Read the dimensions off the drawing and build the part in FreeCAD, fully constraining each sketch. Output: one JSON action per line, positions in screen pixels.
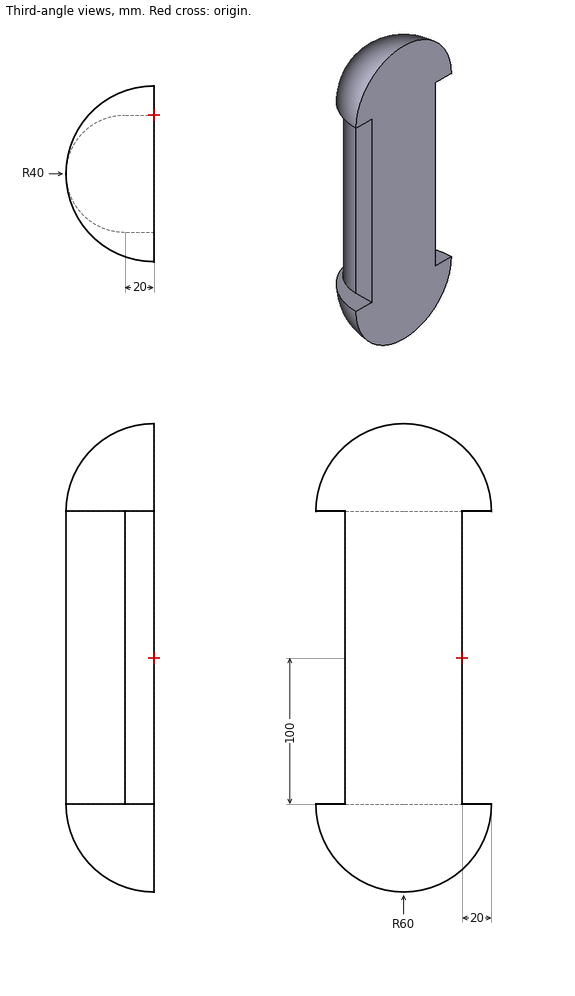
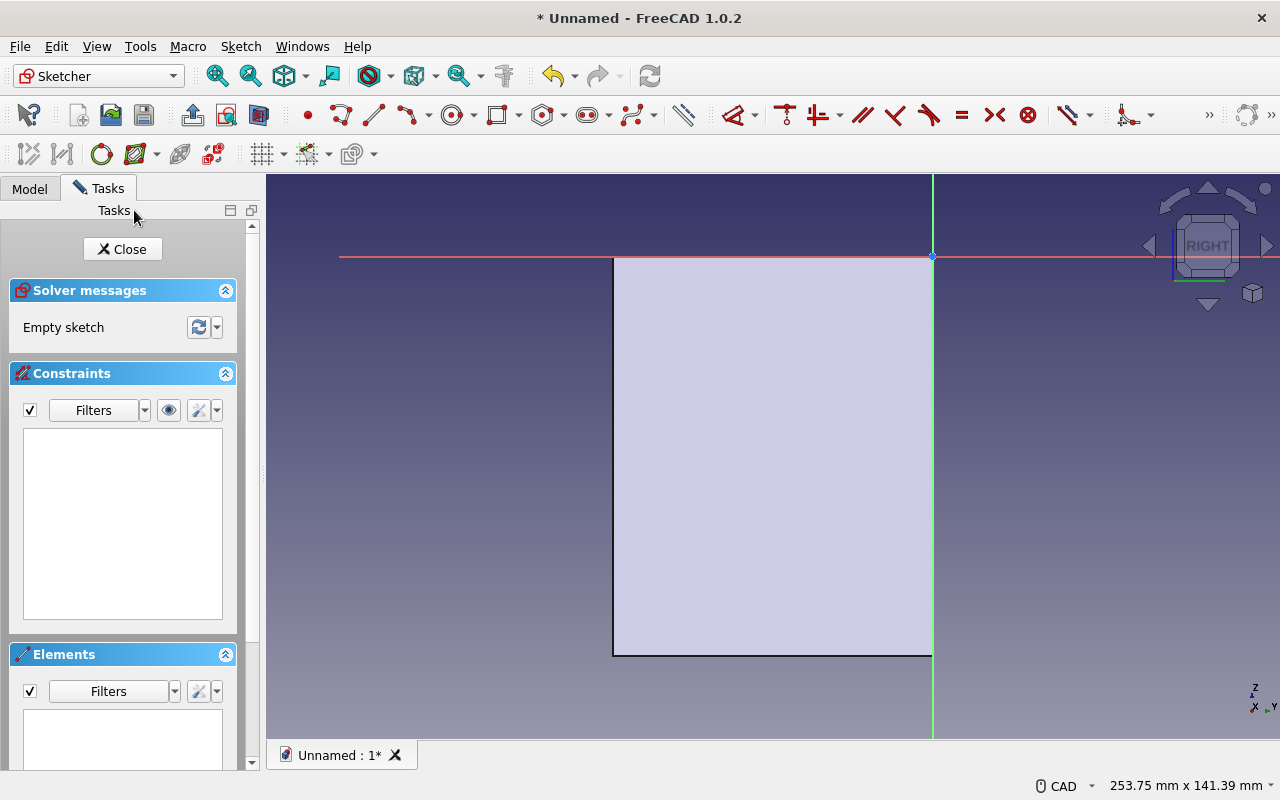
{"action": "scroll", "coordinate": [505, 311], "scroll_direction": "down", "scroll_amount": 3}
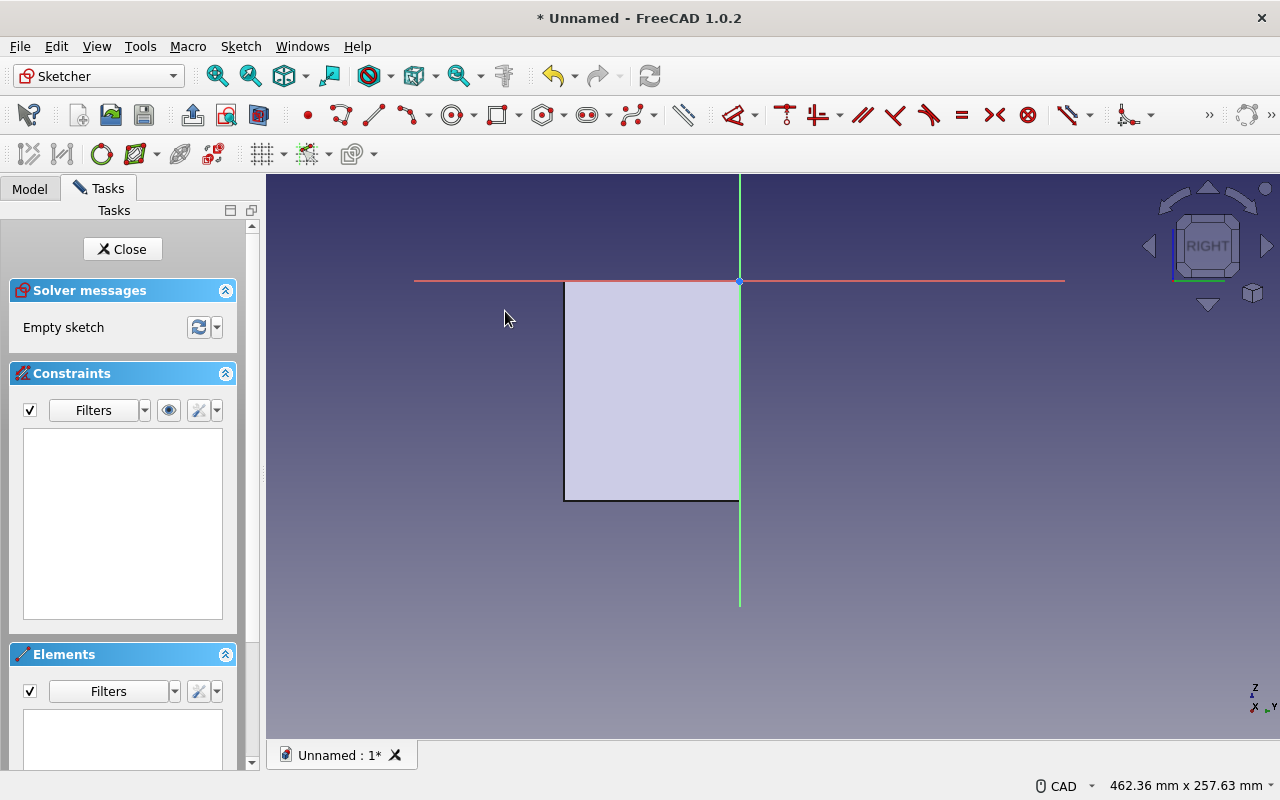
{"action": "key", "text": "g l"}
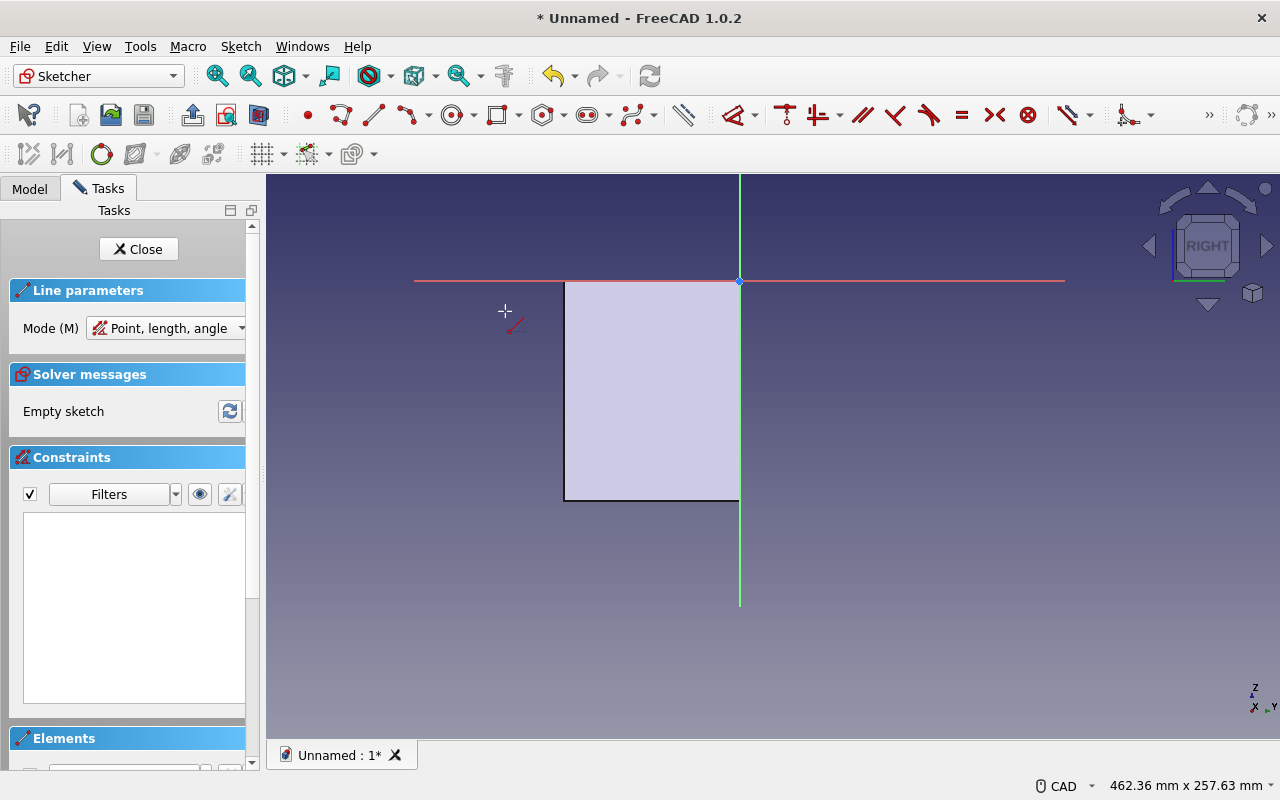
{"action": "left_click", "coordinate": [784, 501]}
{"action": "left_click", "coordinate": [521, 501]}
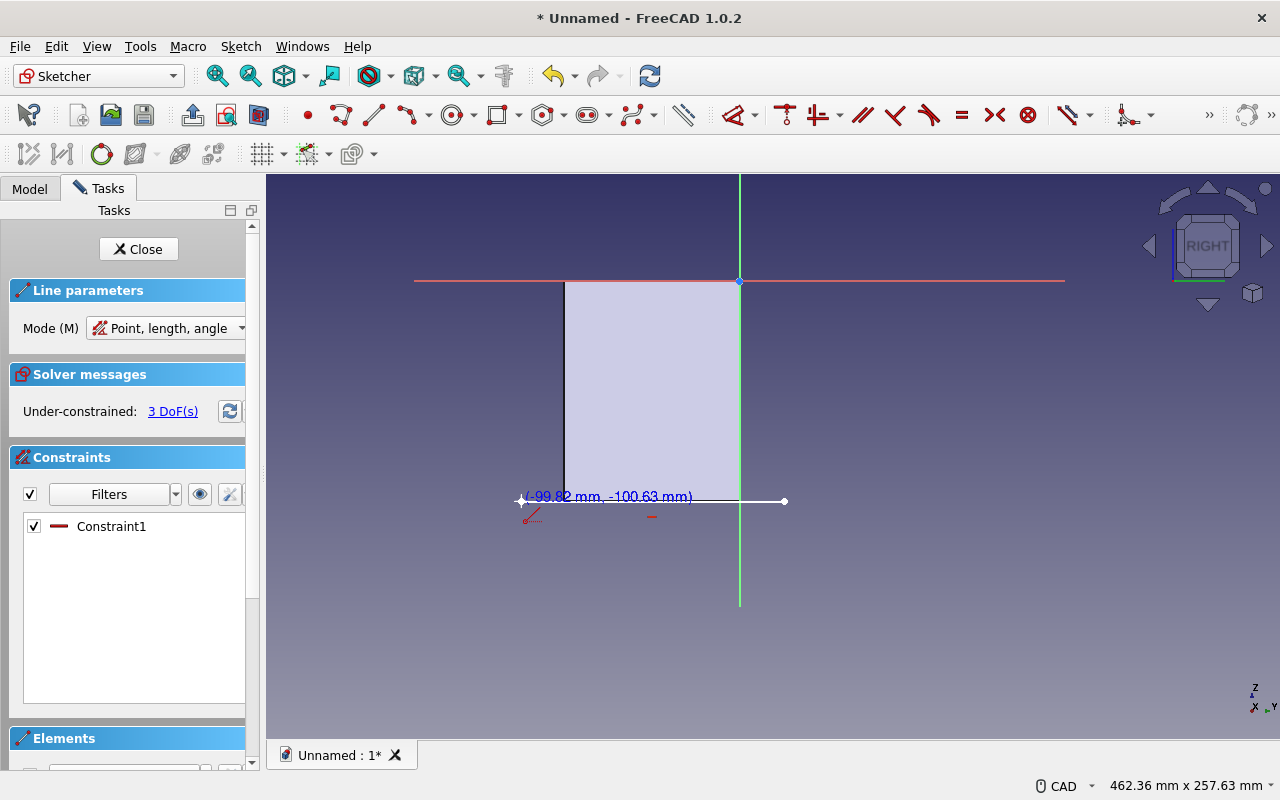
{"action": "left_click", "coordinate": [406, 116]}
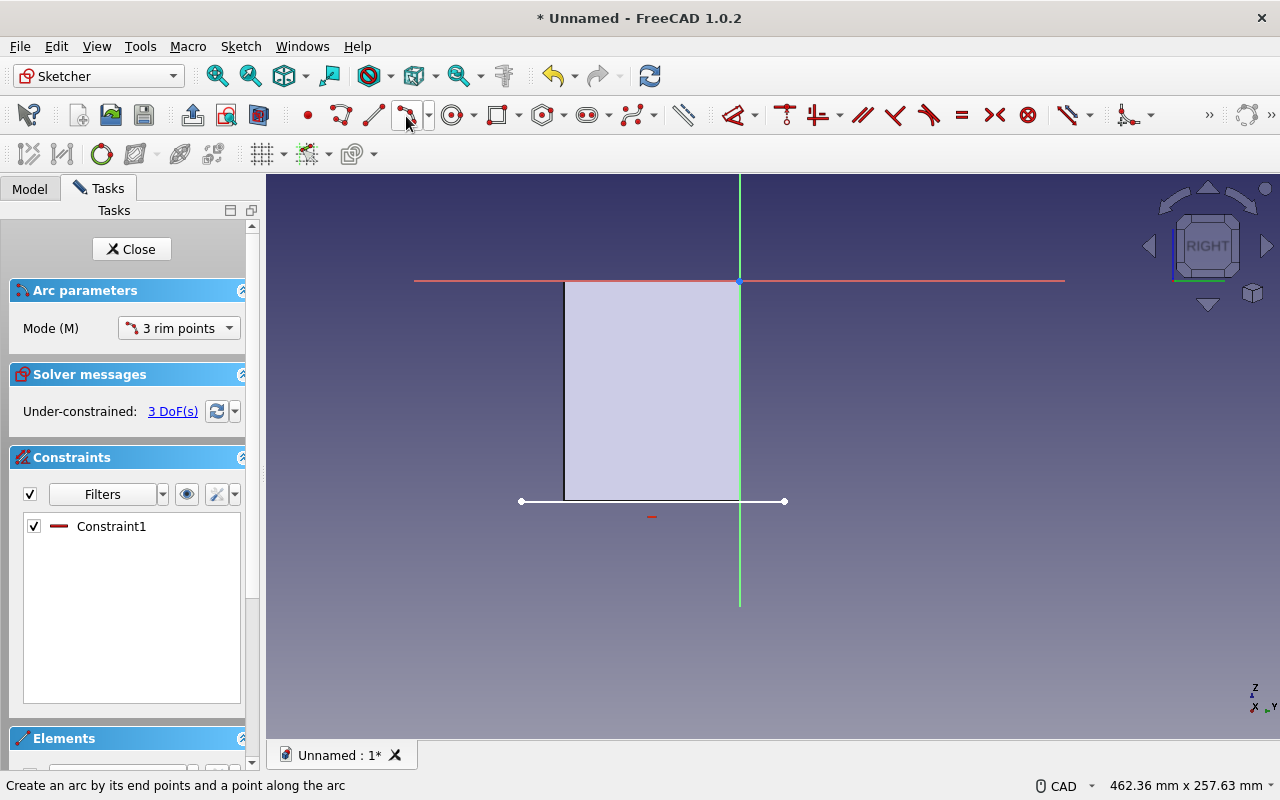
{"action": "left_click", "coordinate": [521, 502]}
{"action": "left_click", "coordinate": [784, 502]}
{"action": "left_click", "coordinate": [652, 632]}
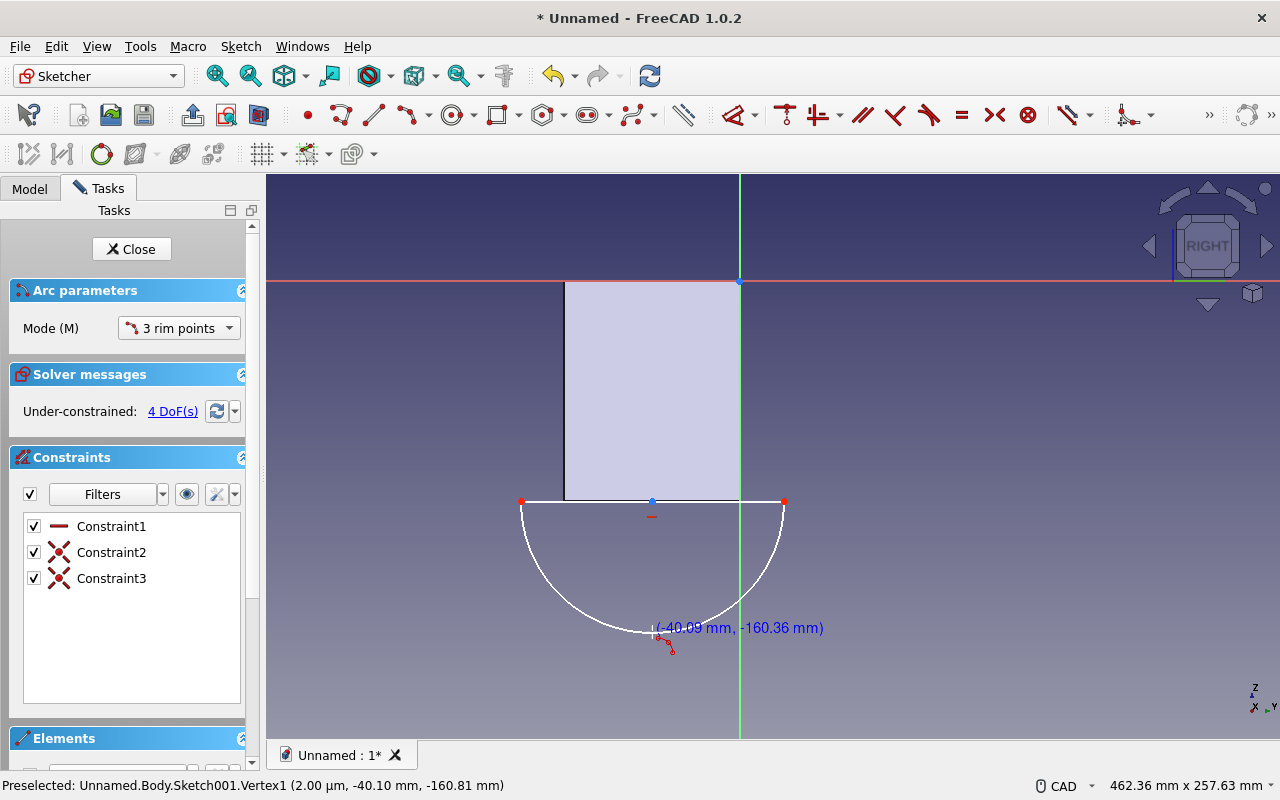
{"action": "left_click", "coordinate": [374, 116]}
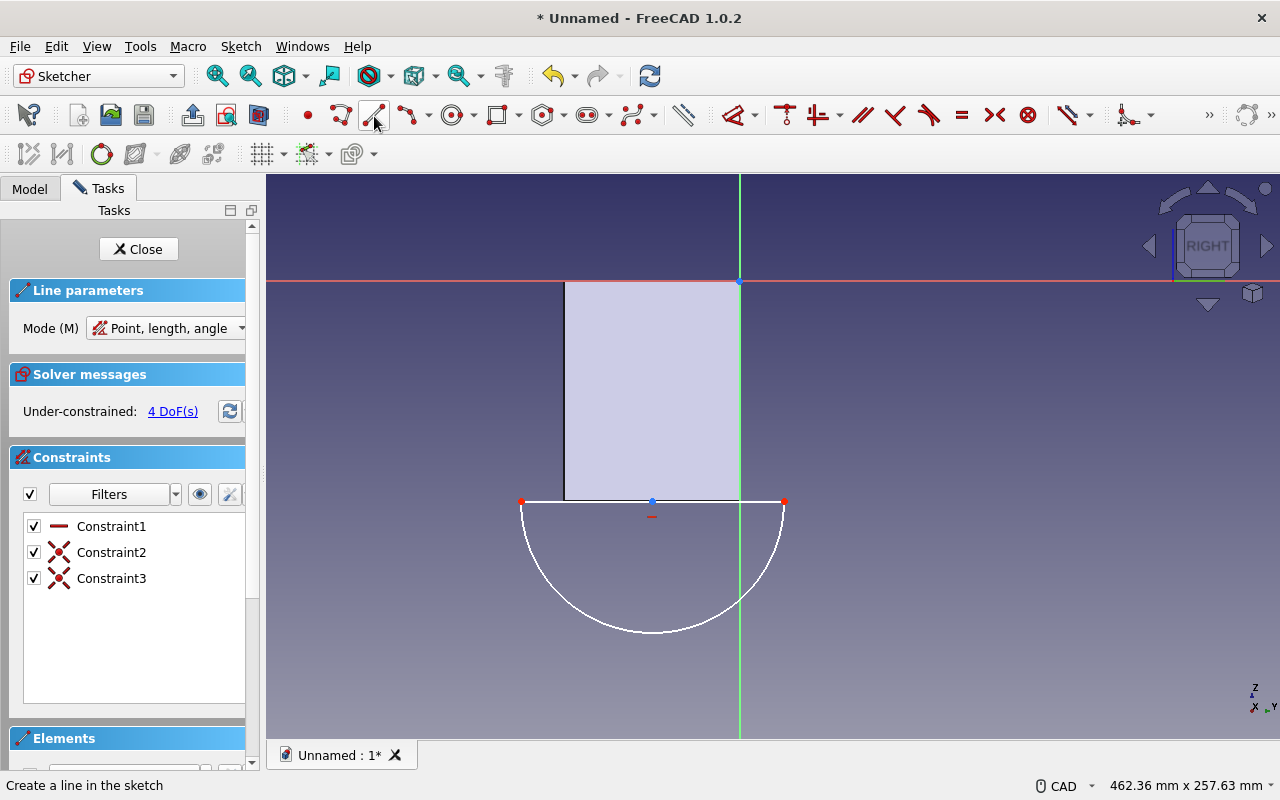
{"action": "left_click", "coordinate": [810, 501]}
{"action": "left_click", "coordinate": [889, 501]}
{"action": "key", "text": "Escape"}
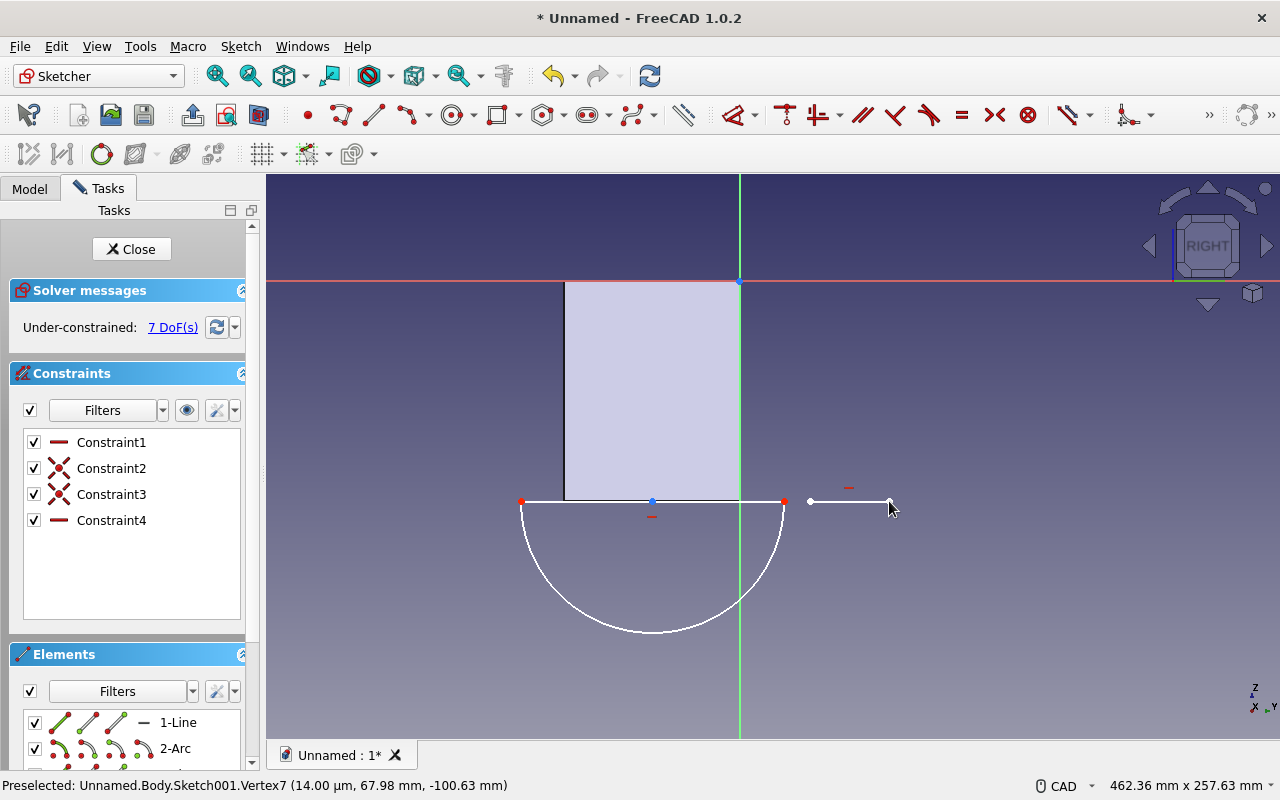
{"action": "left_click", "coordinate": [834, 502]}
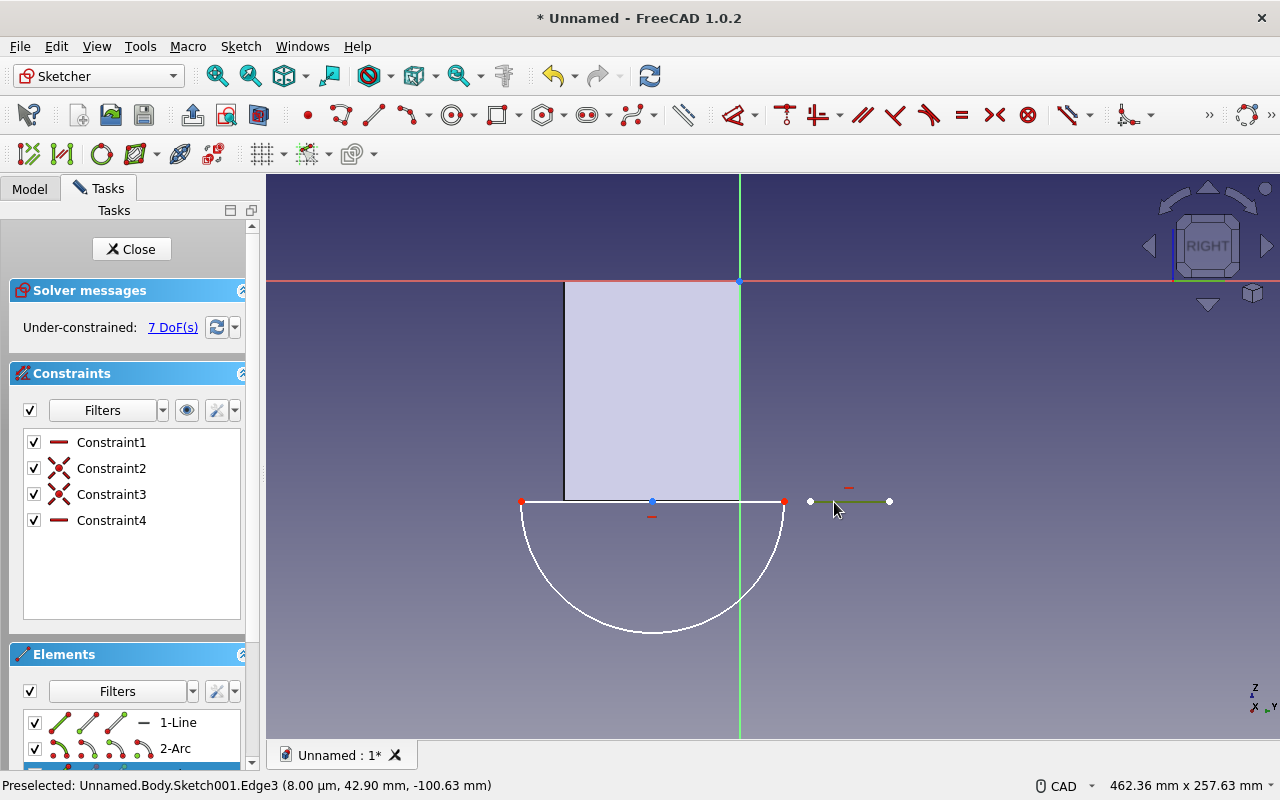
{"action": "key", "text": "g n"}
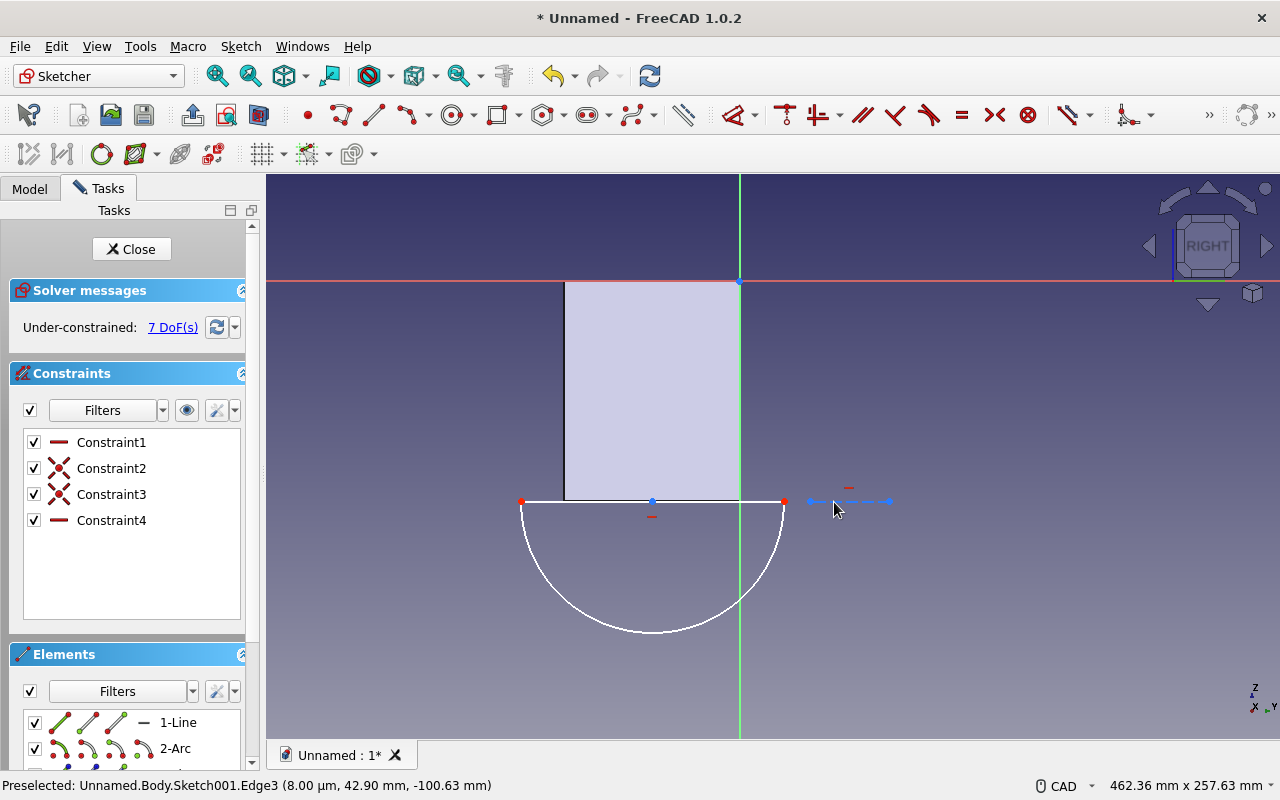
{"action": "key", "text": "d"}